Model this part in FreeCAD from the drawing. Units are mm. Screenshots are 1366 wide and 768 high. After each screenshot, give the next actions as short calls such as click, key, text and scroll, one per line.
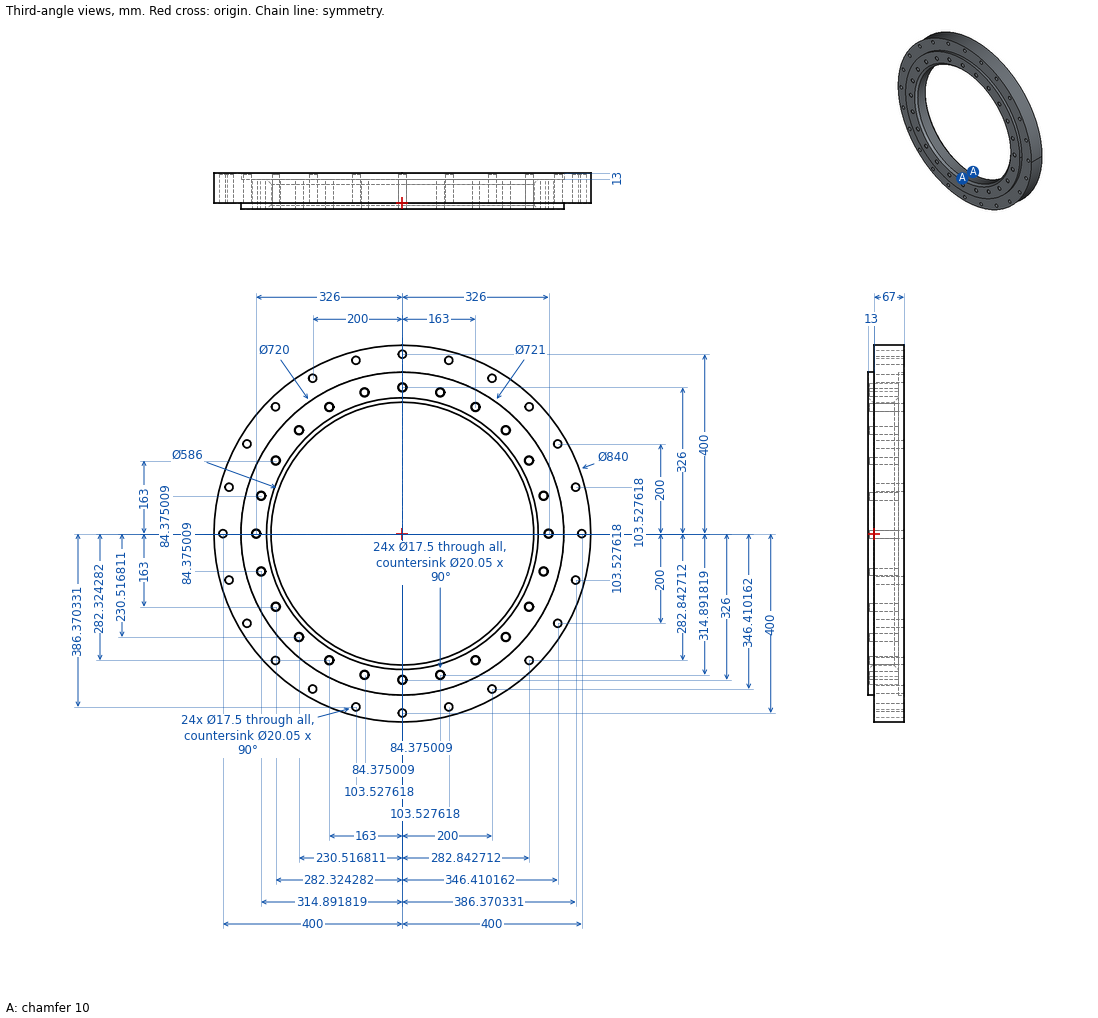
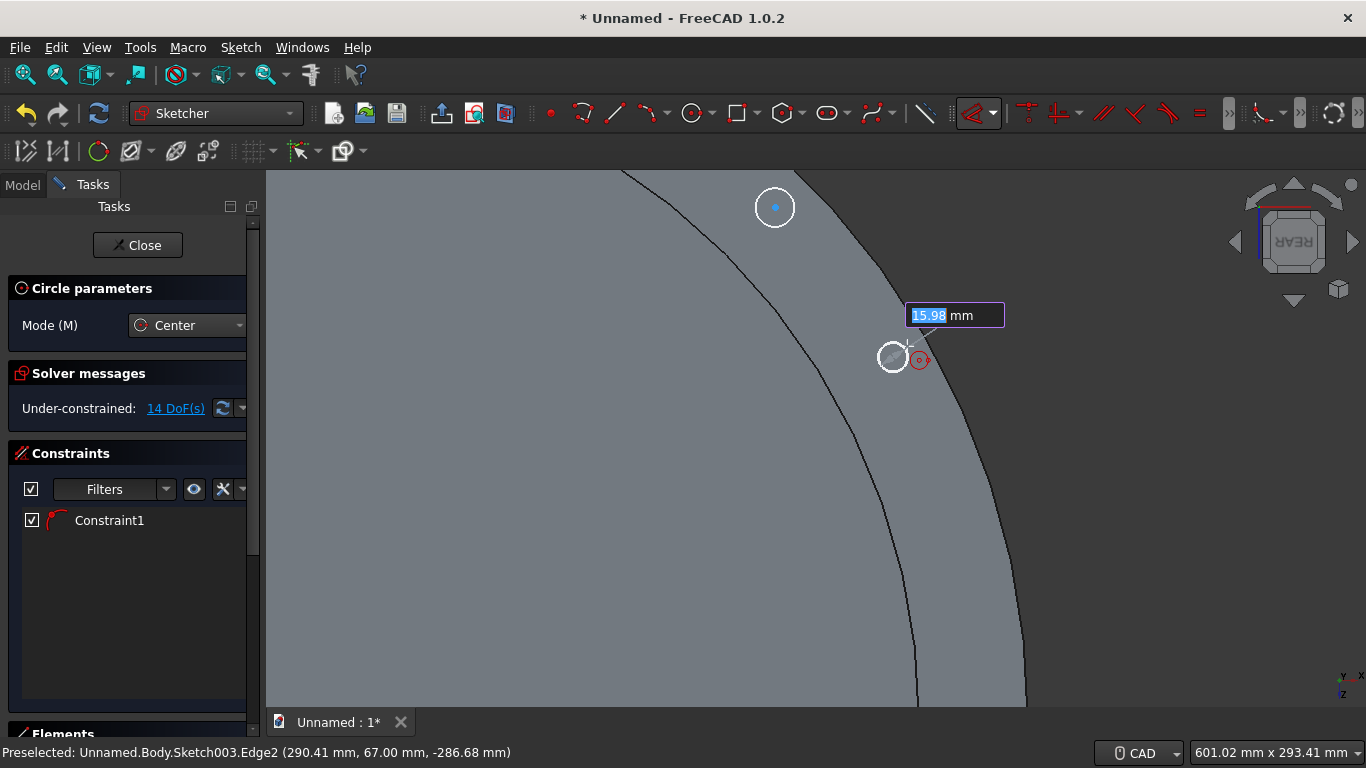
click(904, 344)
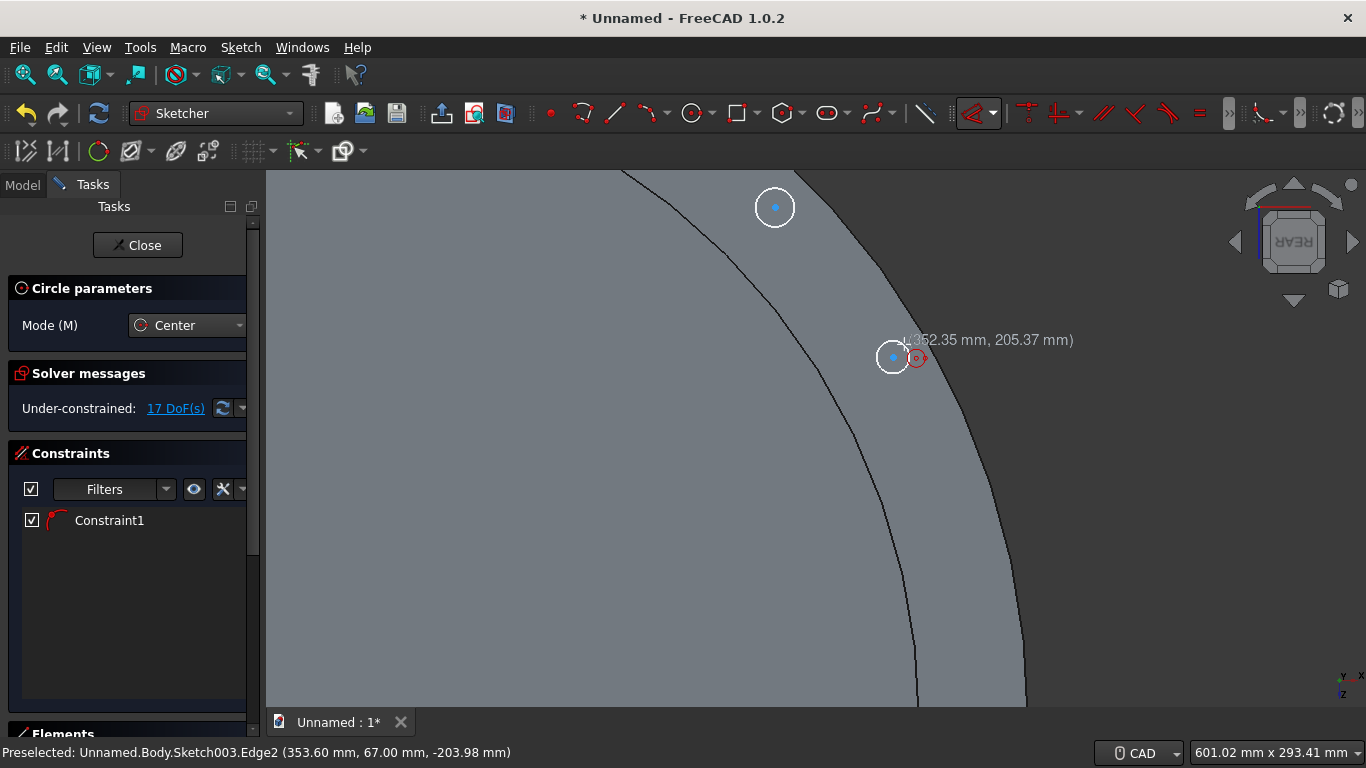
scroll(966, 531, up, 2)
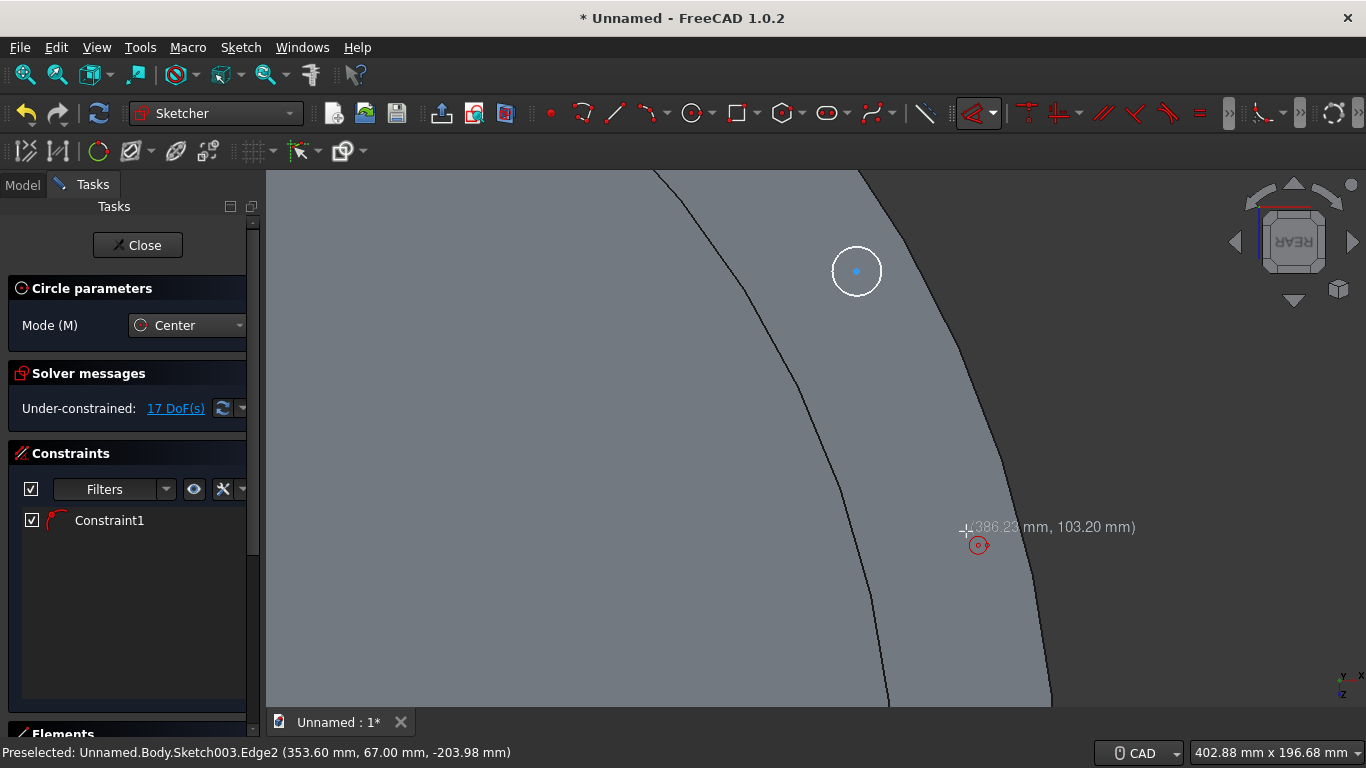
scroll(913, 364, down, 9)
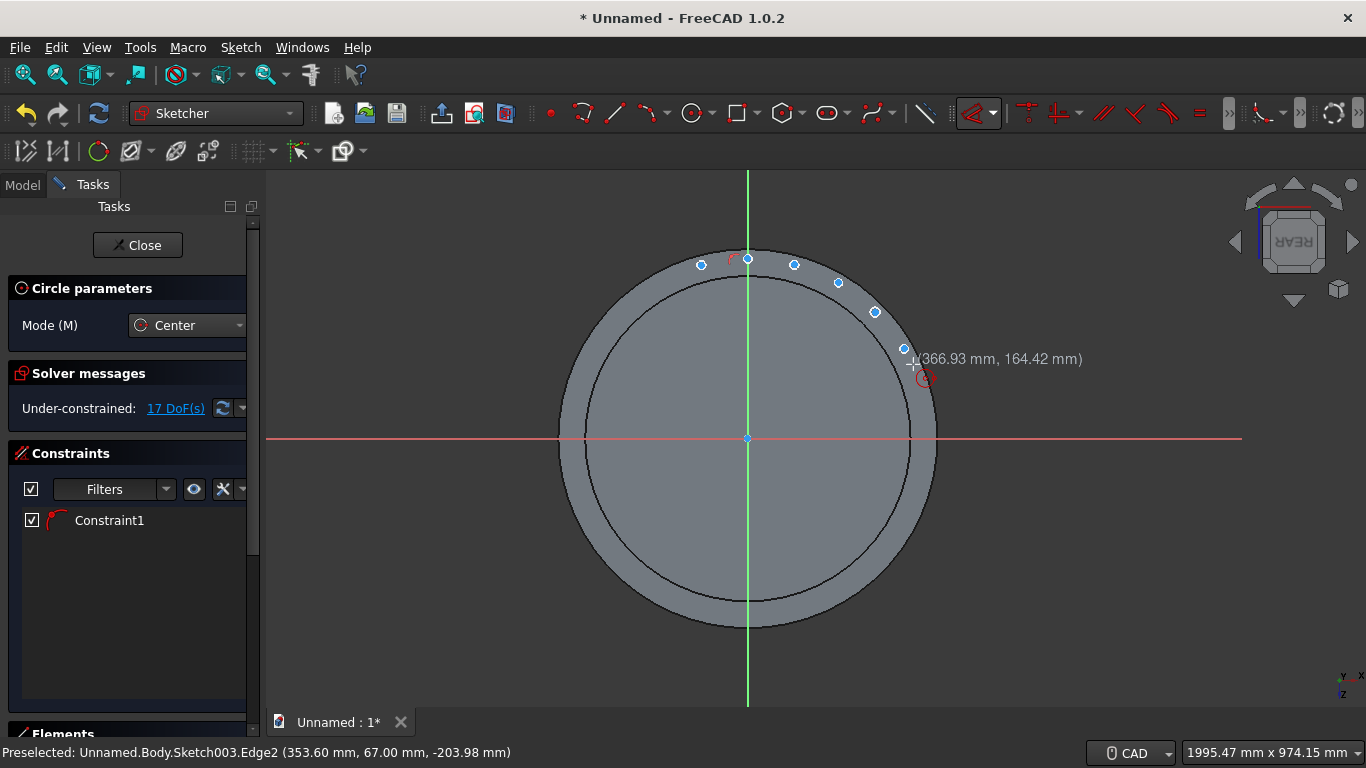
click(922, 392)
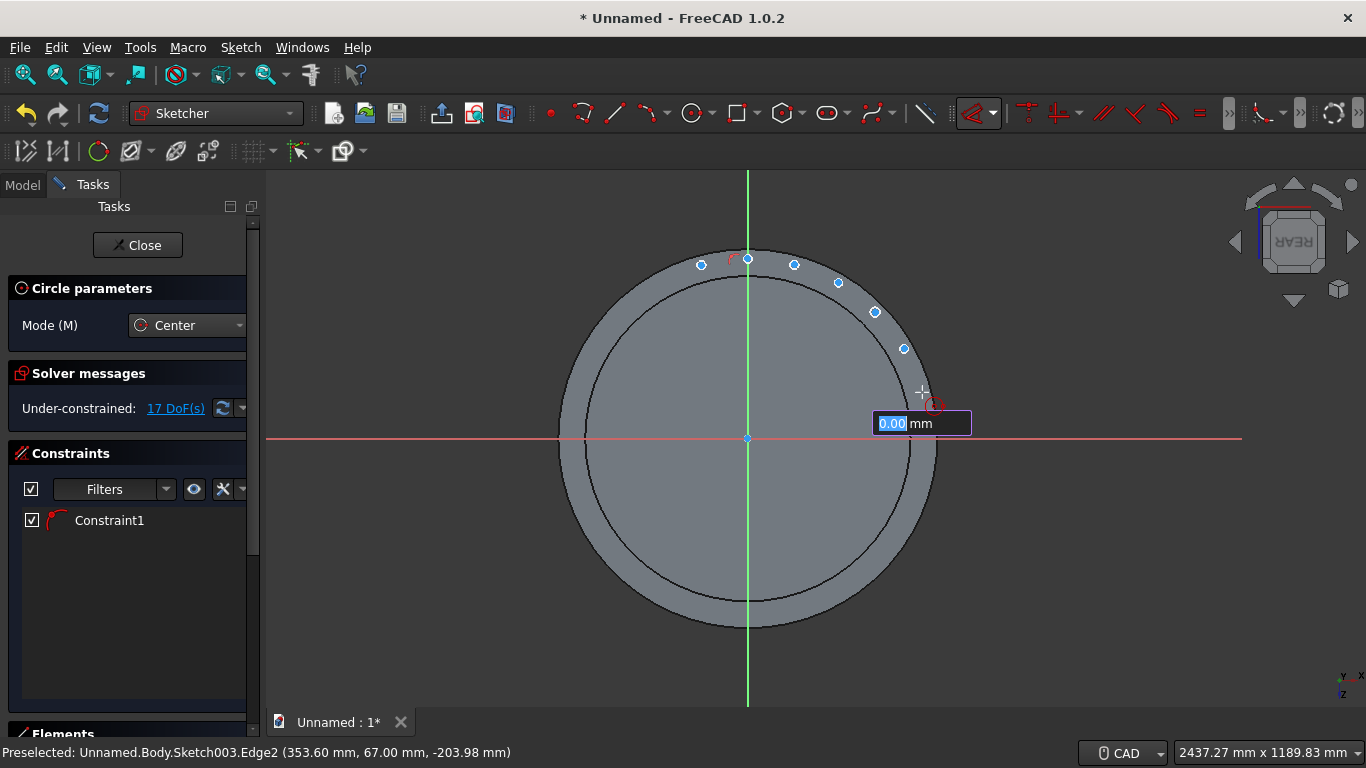
scroll(925, 389, up, 7)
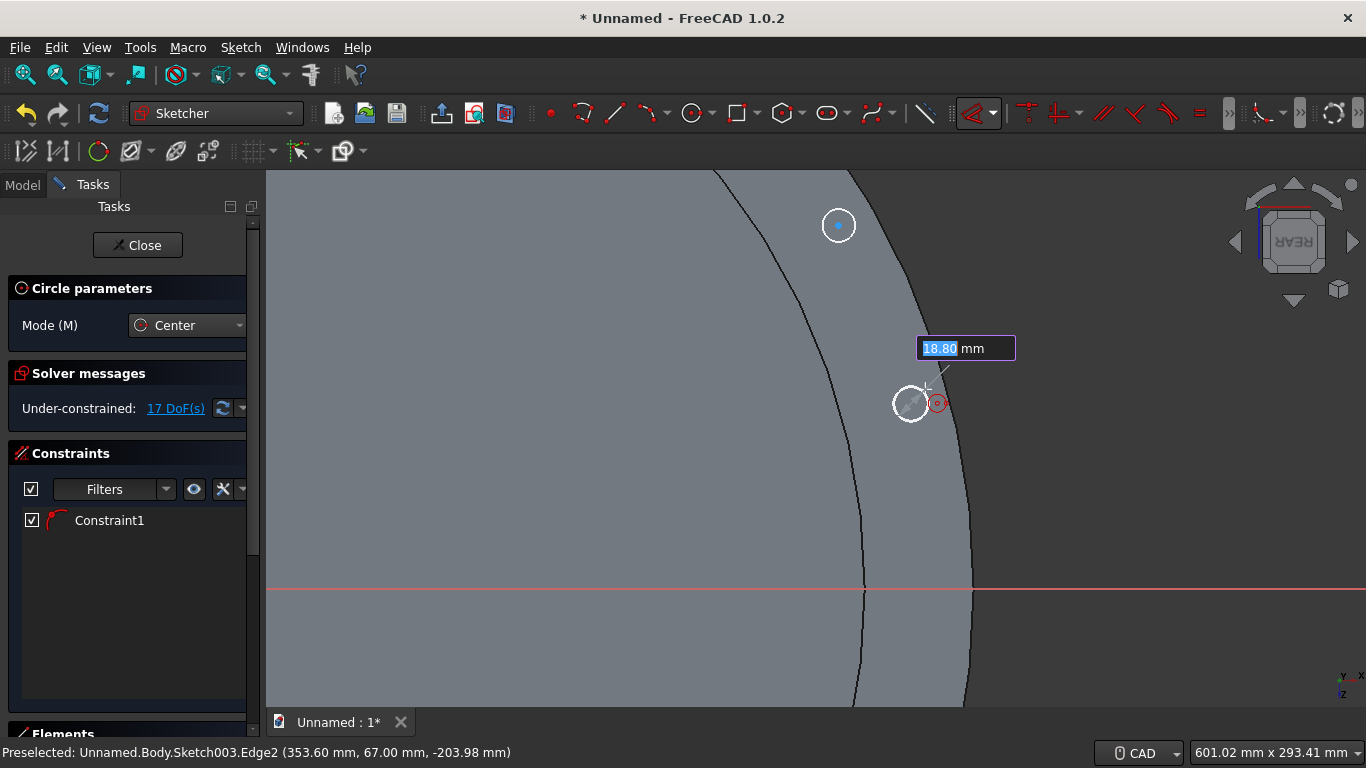
click(923, 388)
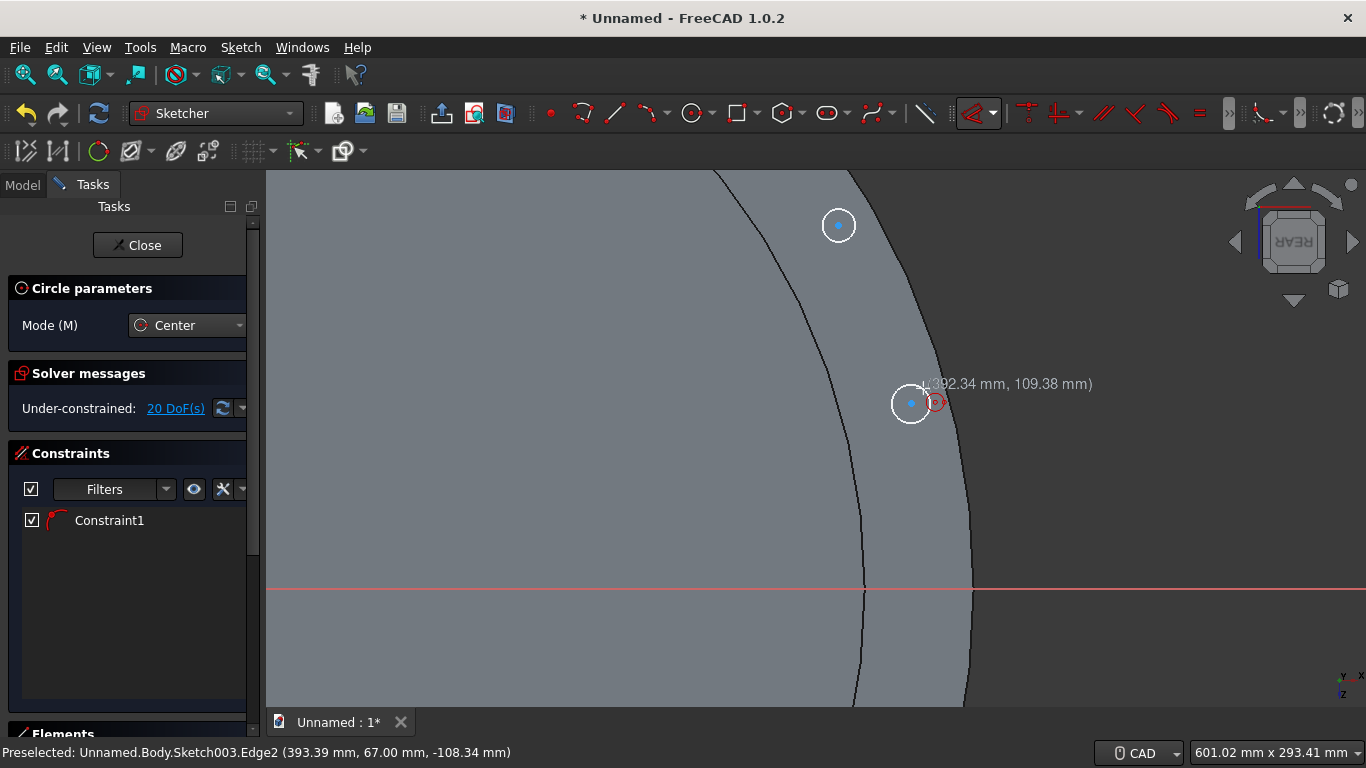
scroll(937, 589, up, 2)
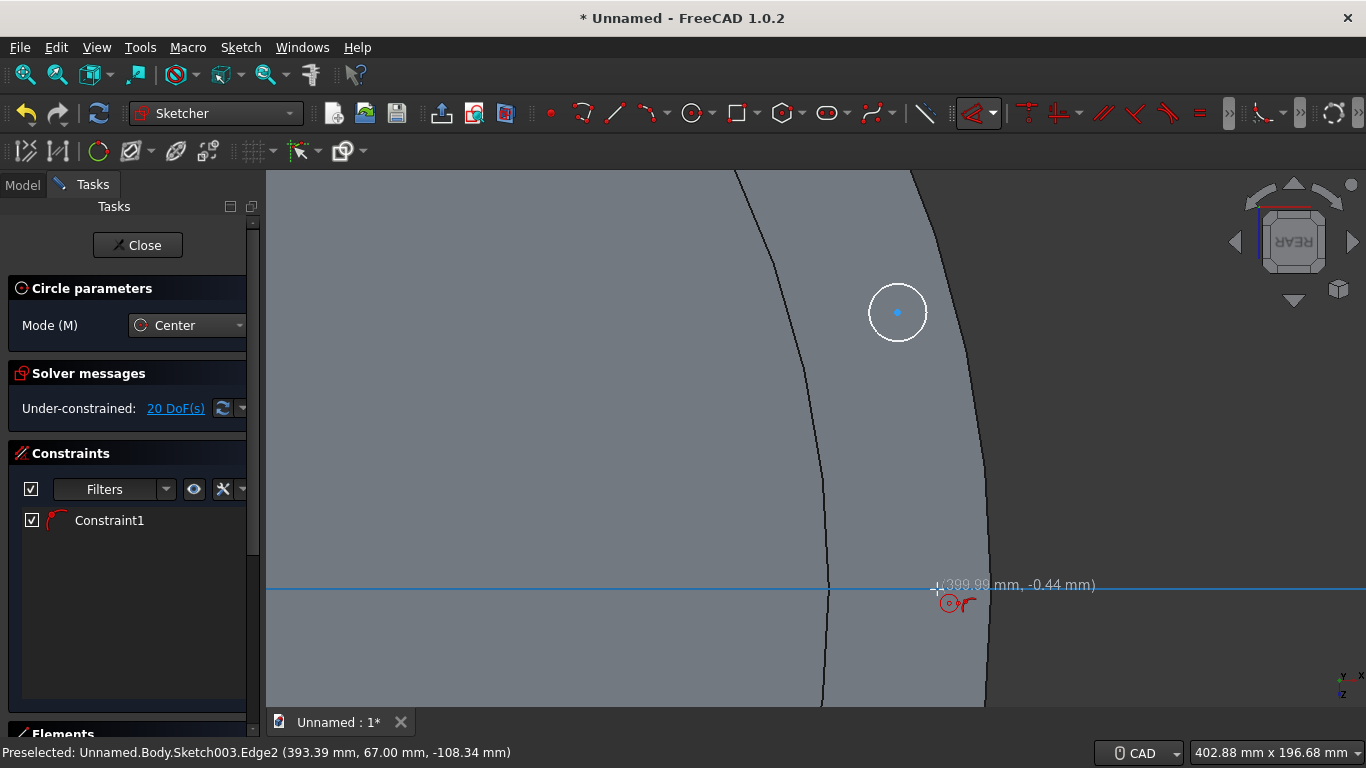
scroll(926, 409, down, 9)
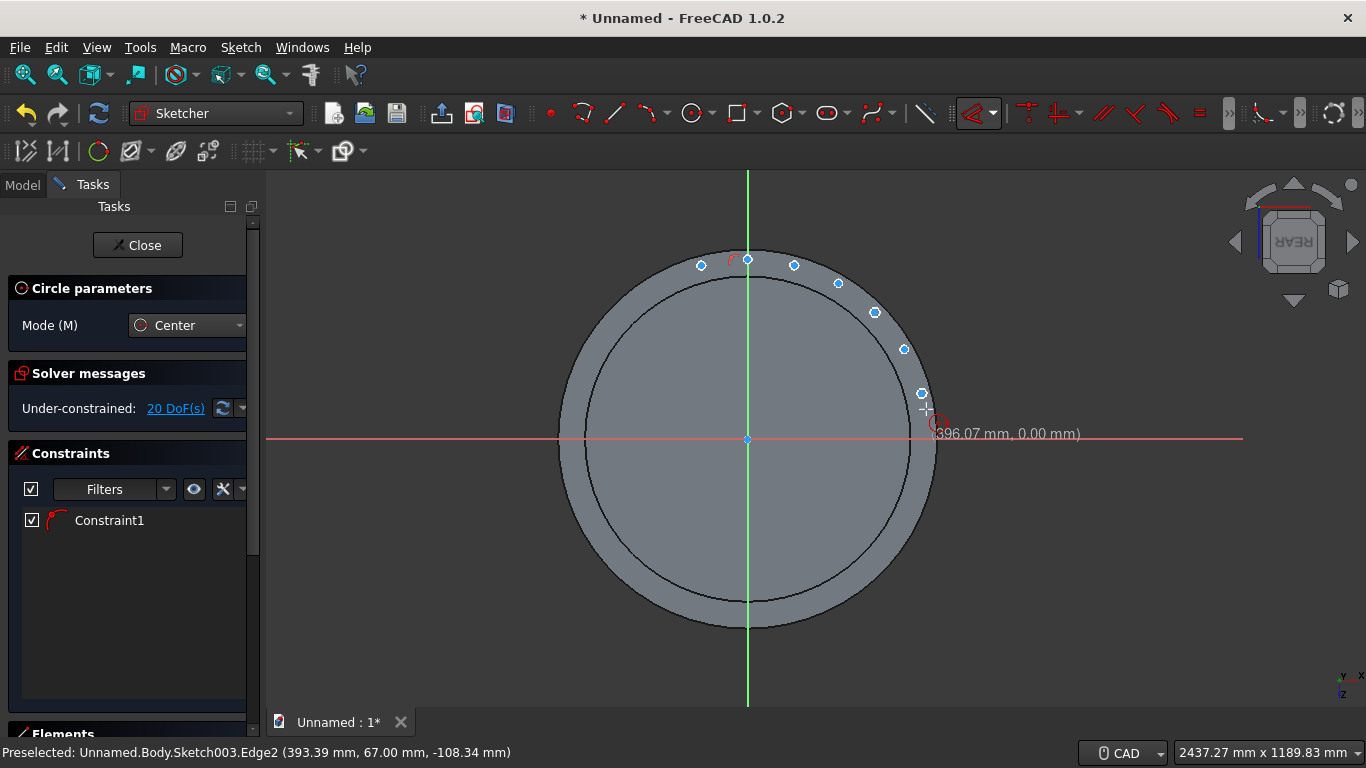
click(928, 439)